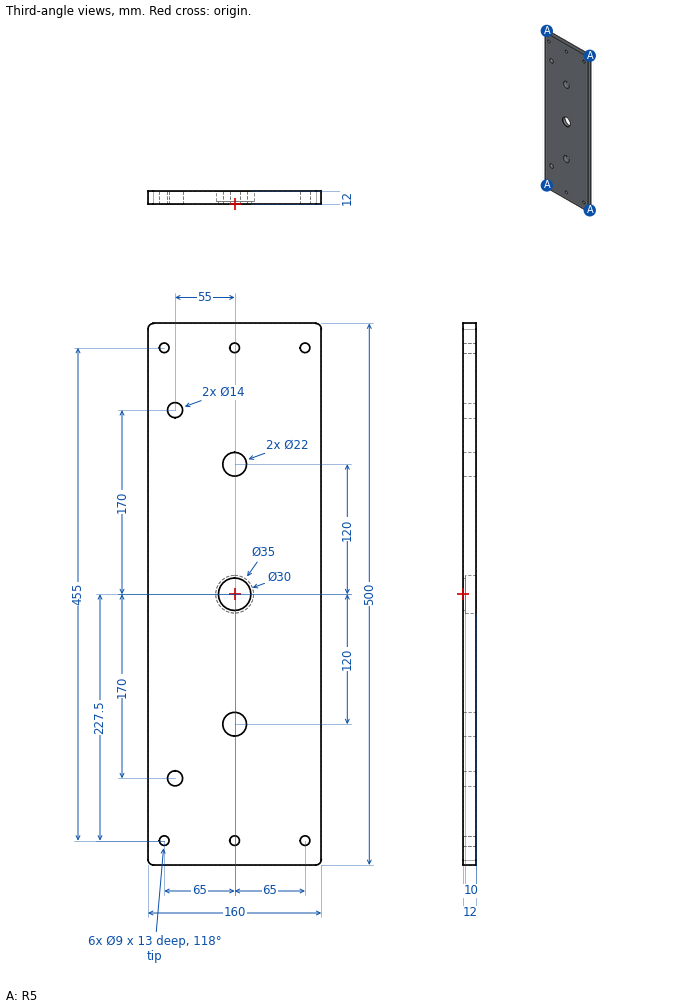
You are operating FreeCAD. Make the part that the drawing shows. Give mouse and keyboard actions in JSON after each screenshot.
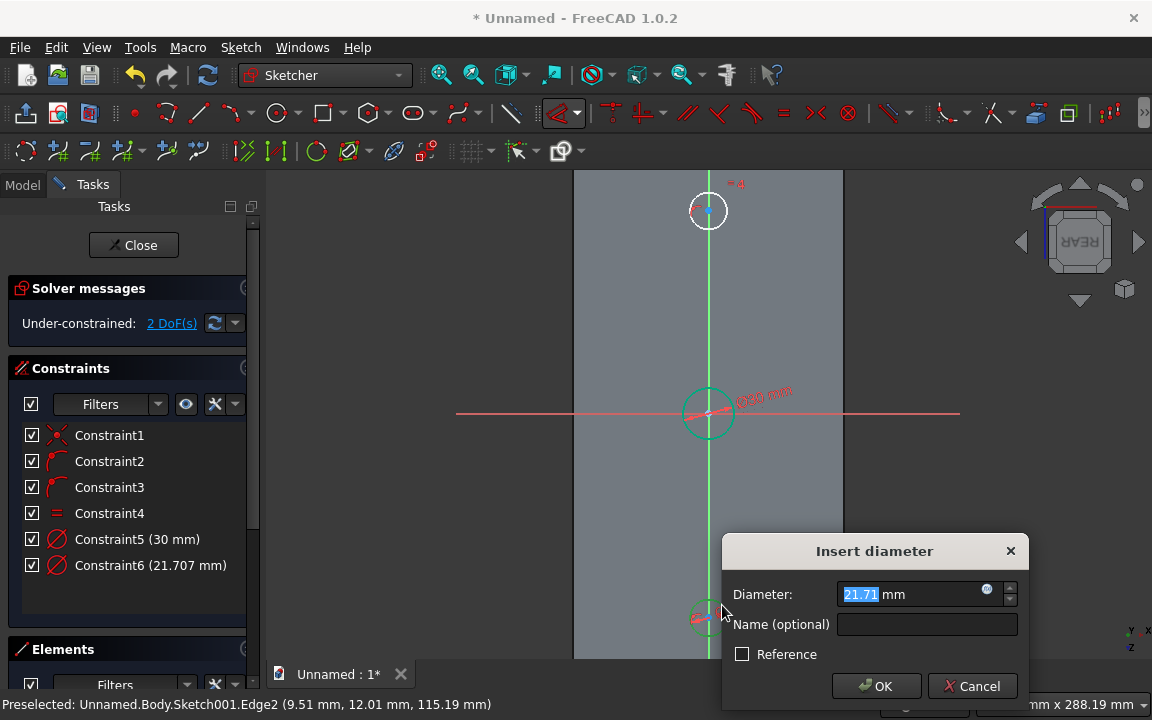
{"action": "type", "text": "22"}
{"action": "key", "text": "Return"}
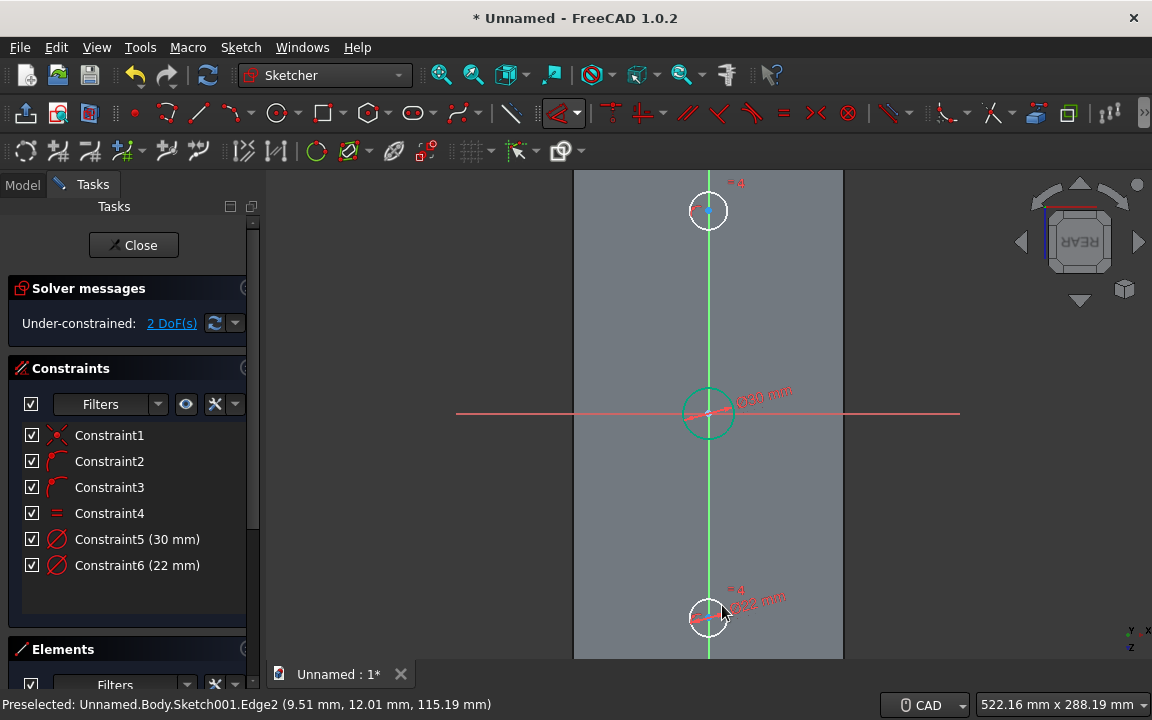
{"action": "left_click", "coordinate": [709, 618]}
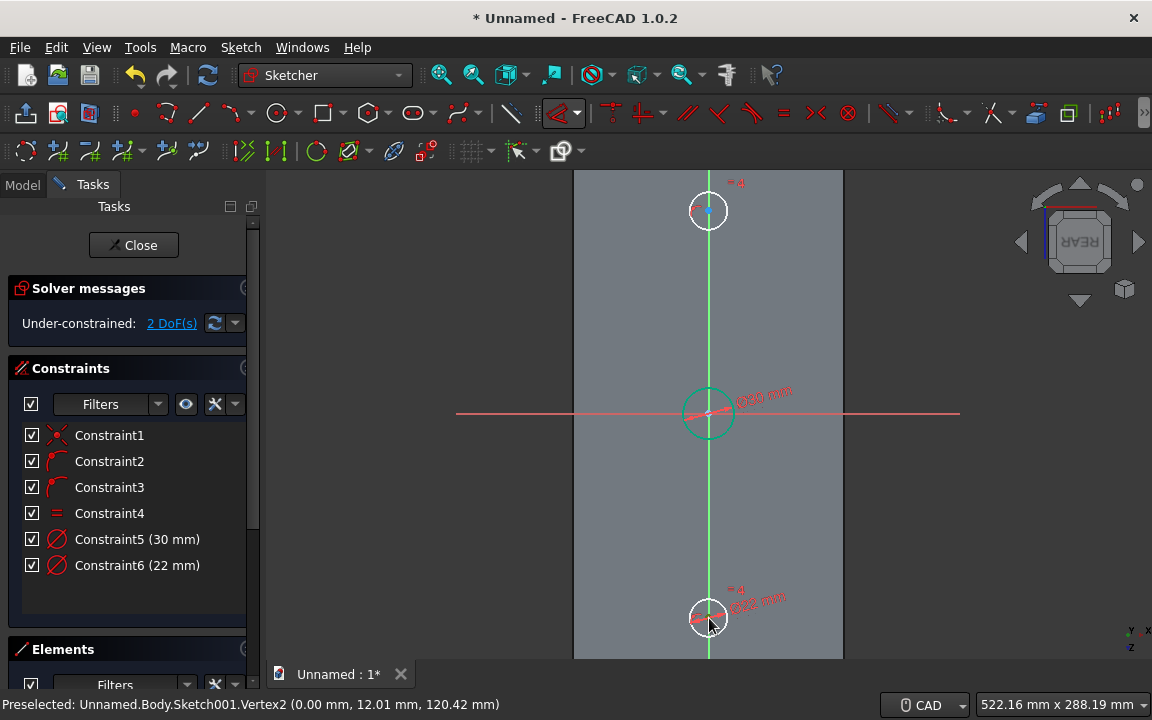
{"action": "left_click", "coordinate": [580, 114]}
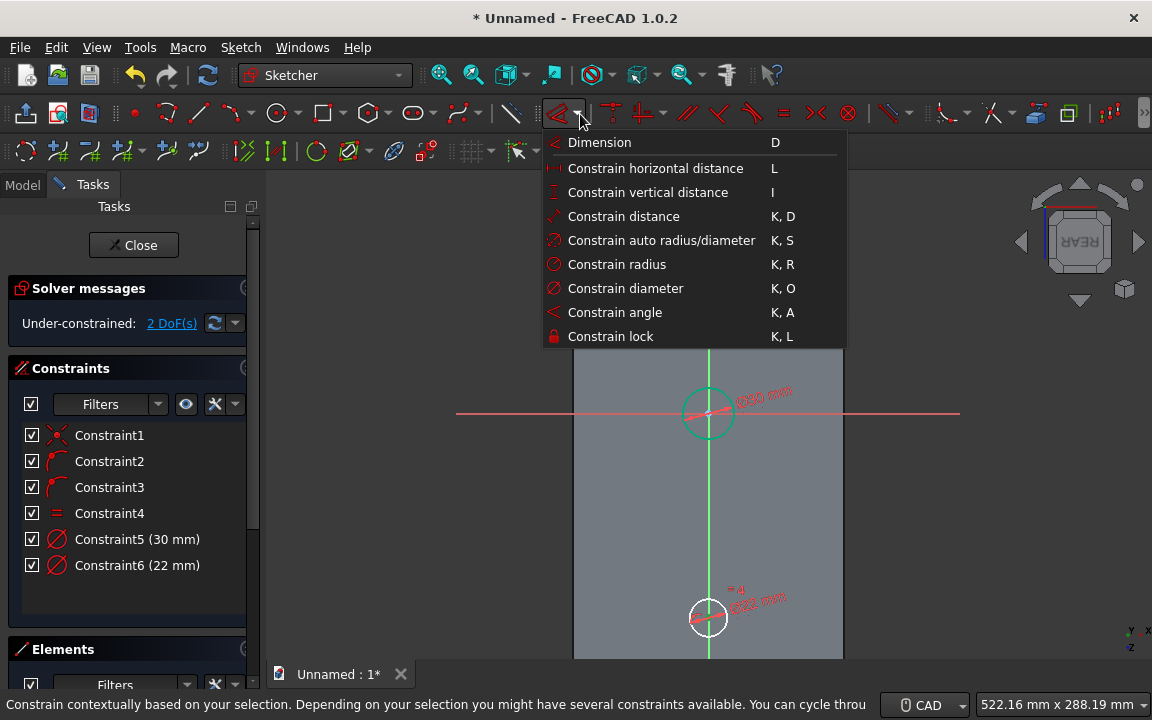
{"action": "left_click", "coordinate": [695, 192]}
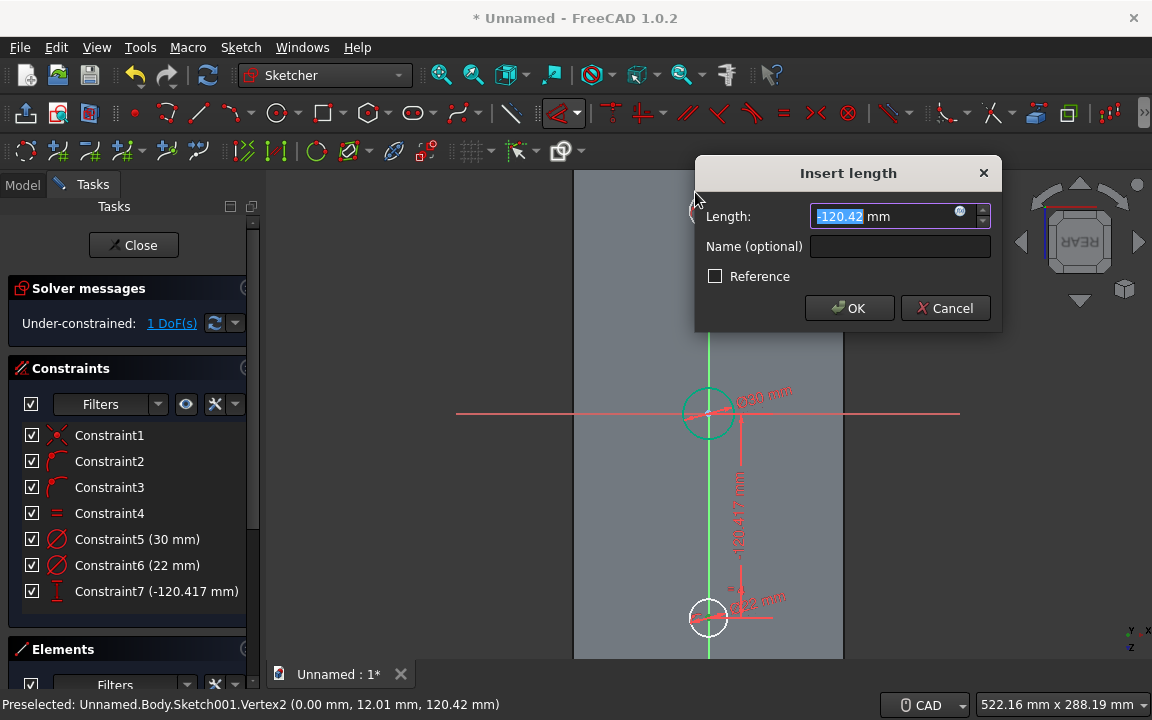
{"action": "type", "text": "-120"}
{"action": "key", "text": "Return"}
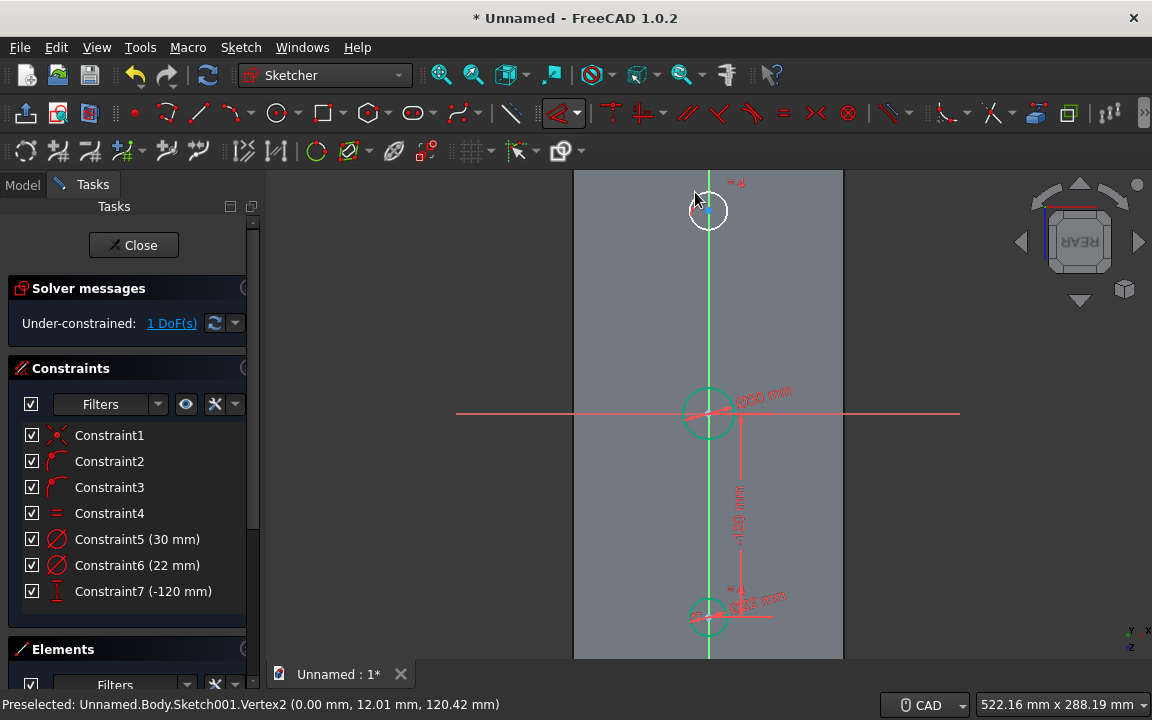
{"action": "left_click", "coordinate": [709, 211]}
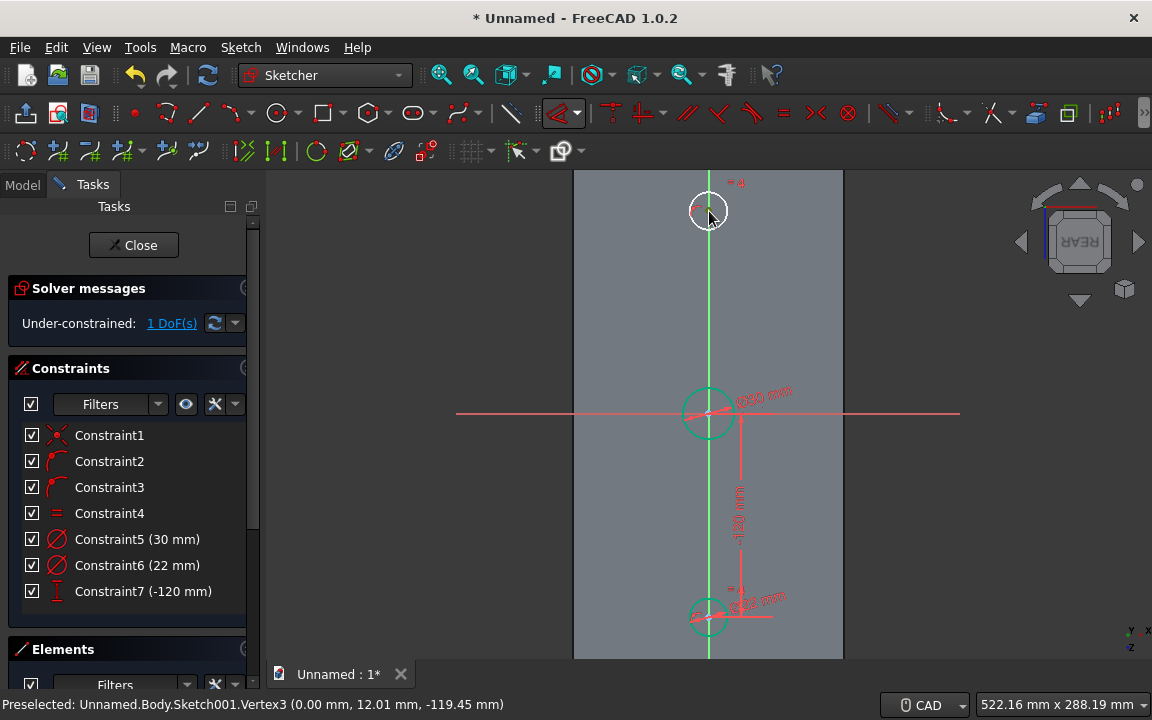
{"action": "left_click", "coordinate": [580, 114]}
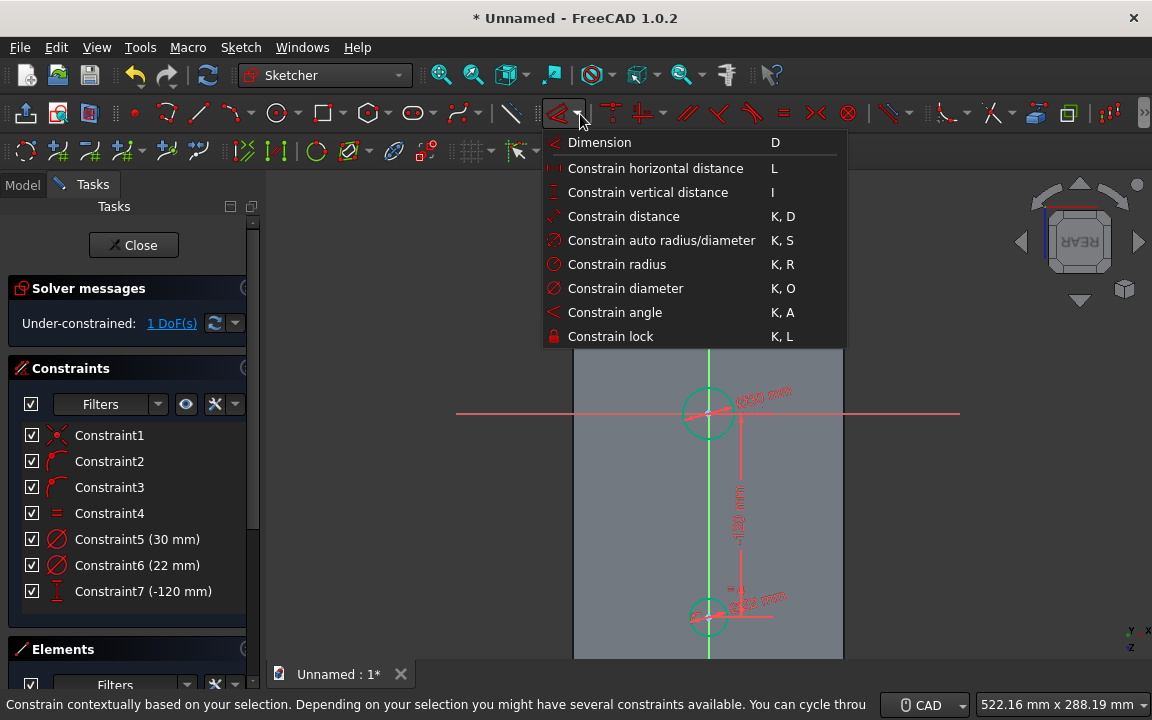
{"action": "left_click", "coordinate": [695, 192]}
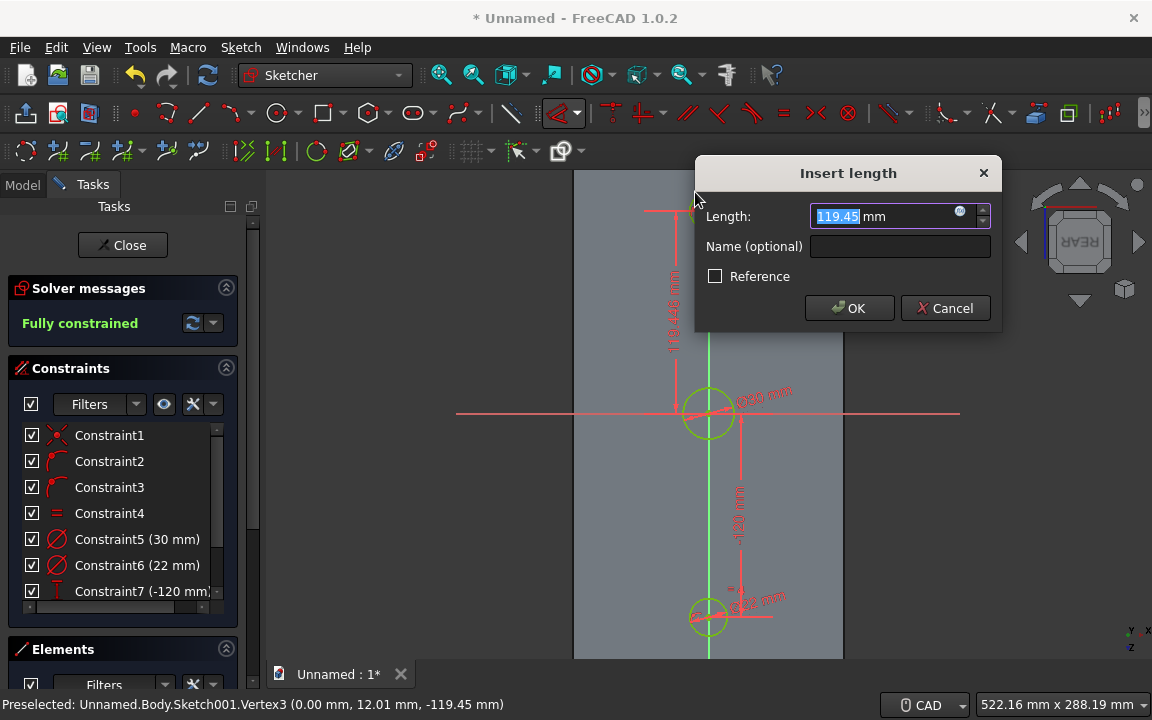
{"action": "type", "text": "120"}
{"action": "key", "text": "Return"}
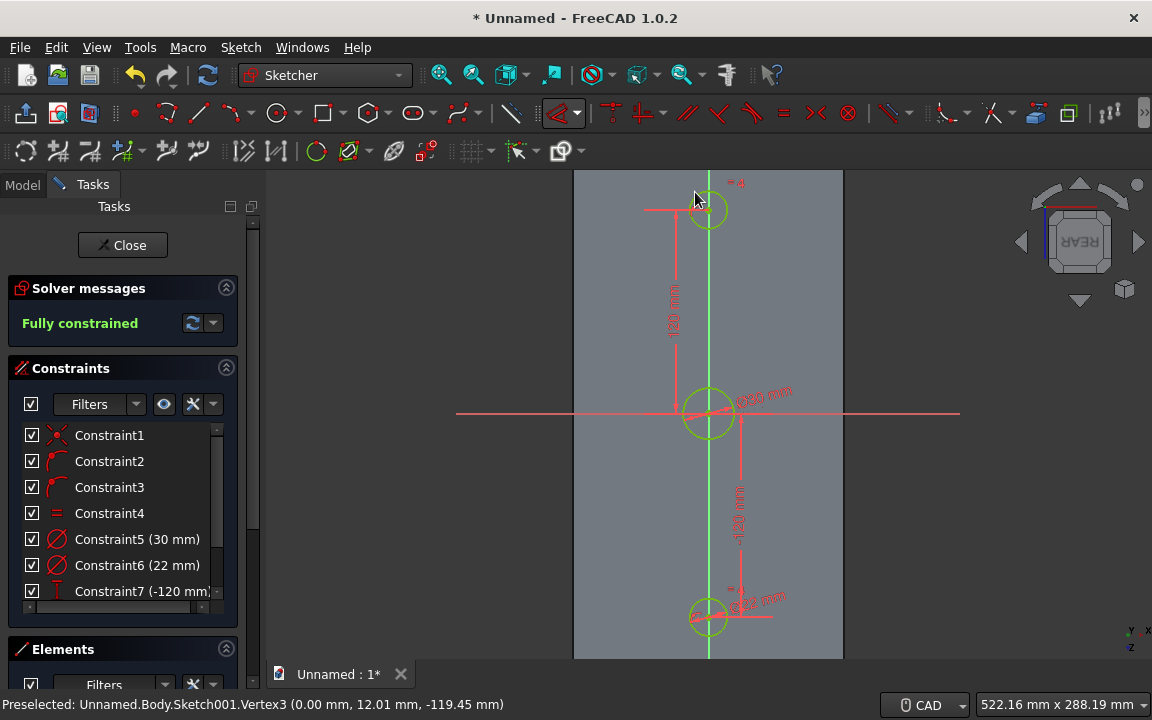
{"action": "left_click", "coordinate": [123, 245]}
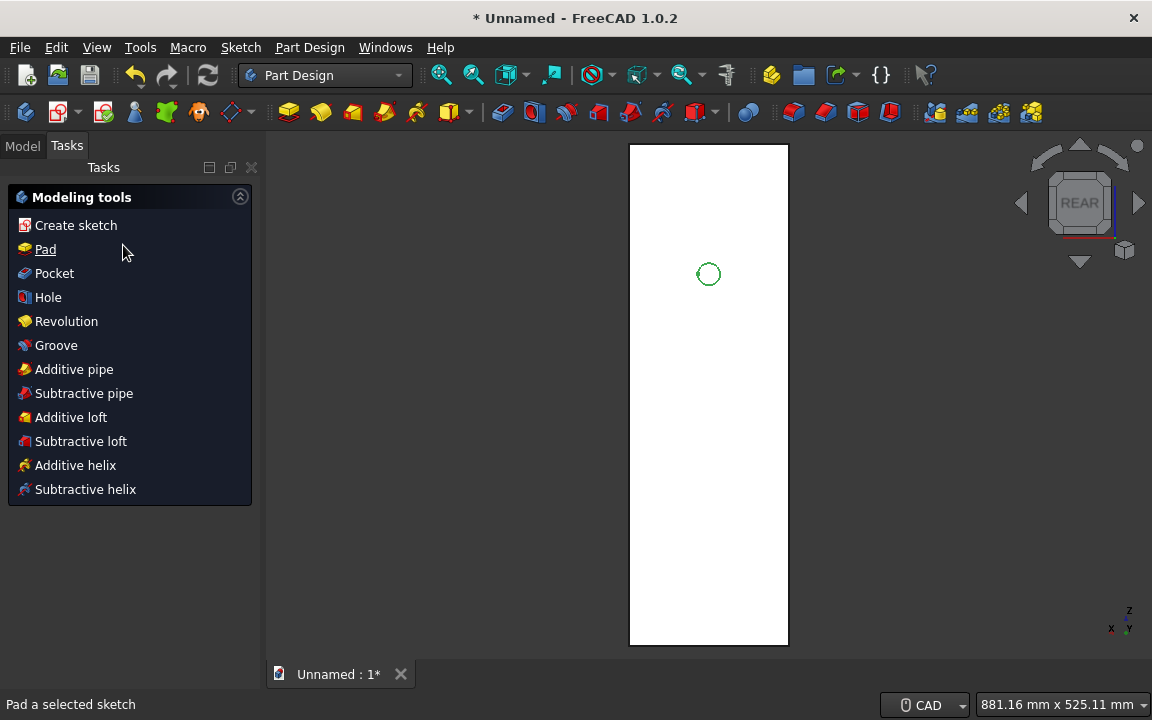
{"action": "left_click", "coordinate": [504, 112]}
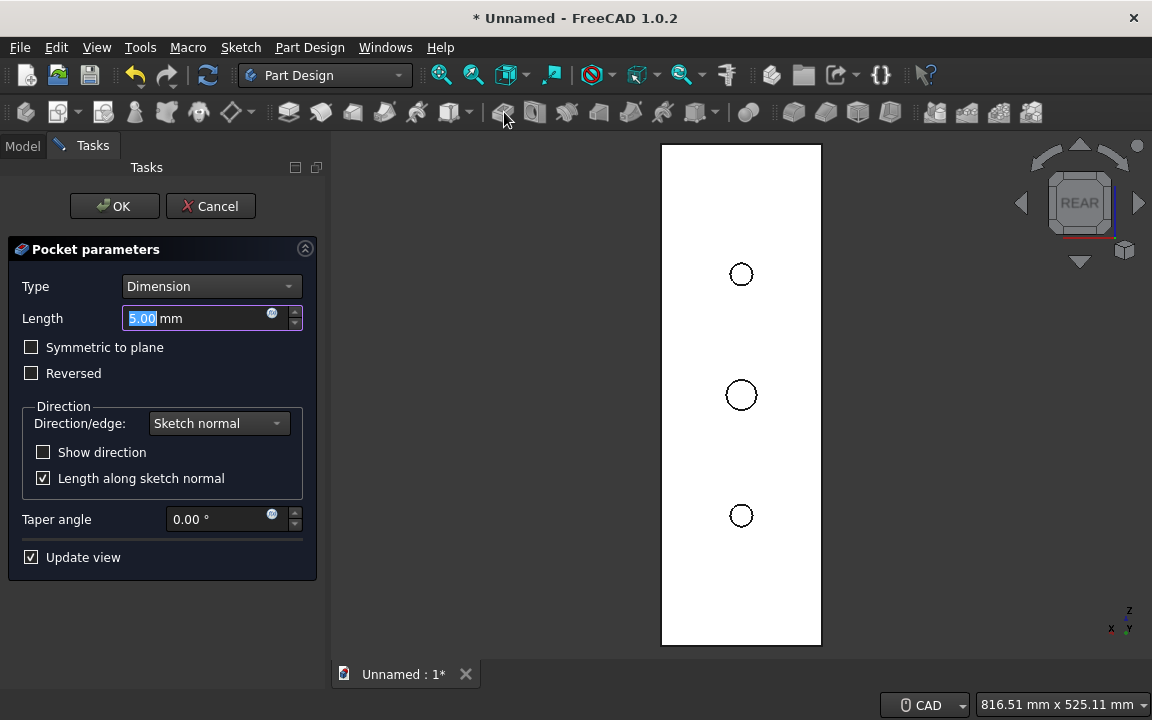
{"action": "type", "text": "12"}
{"action": "key", "text": "Tab"}